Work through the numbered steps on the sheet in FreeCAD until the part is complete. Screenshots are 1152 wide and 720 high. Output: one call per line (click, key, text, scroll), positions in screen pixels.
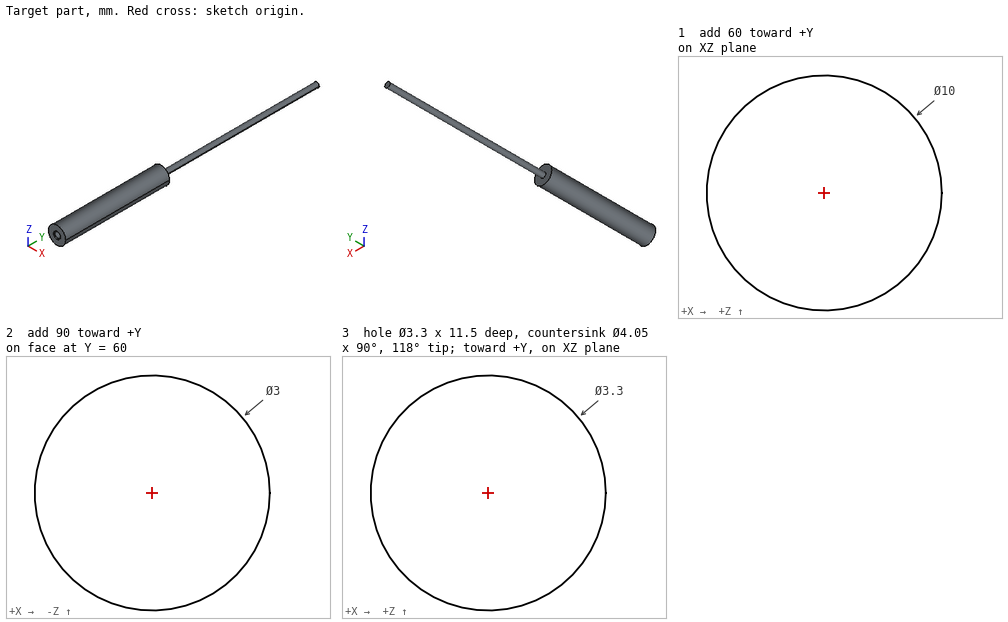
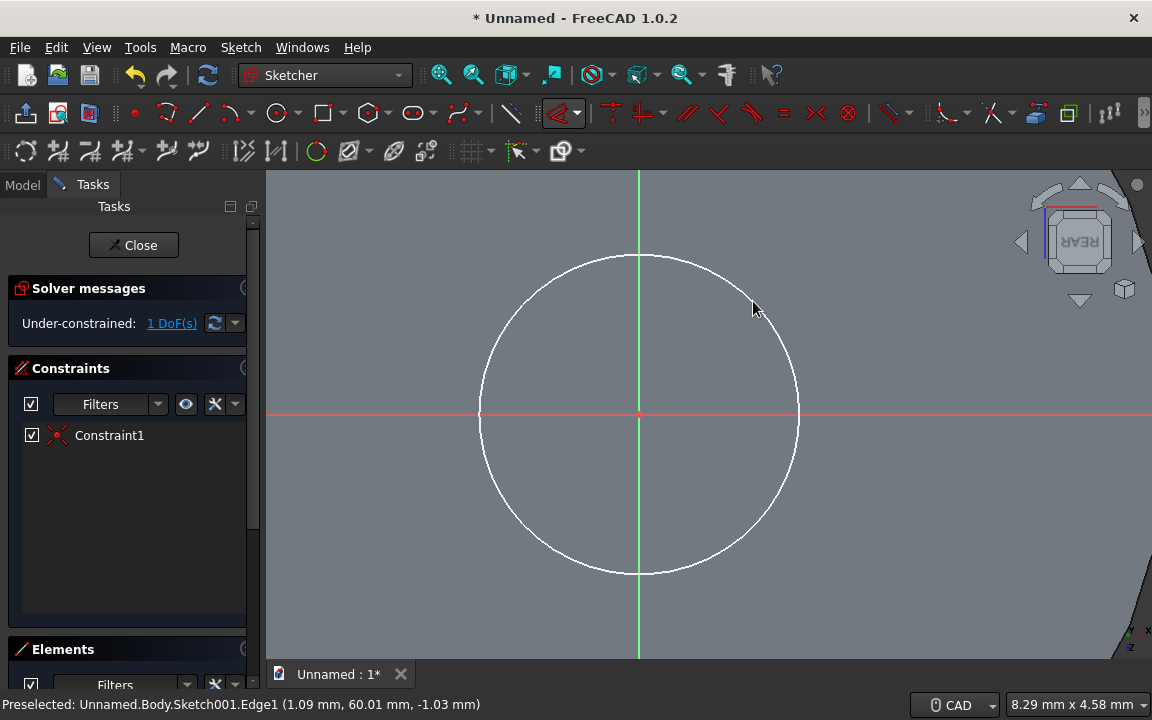
click(752, 301)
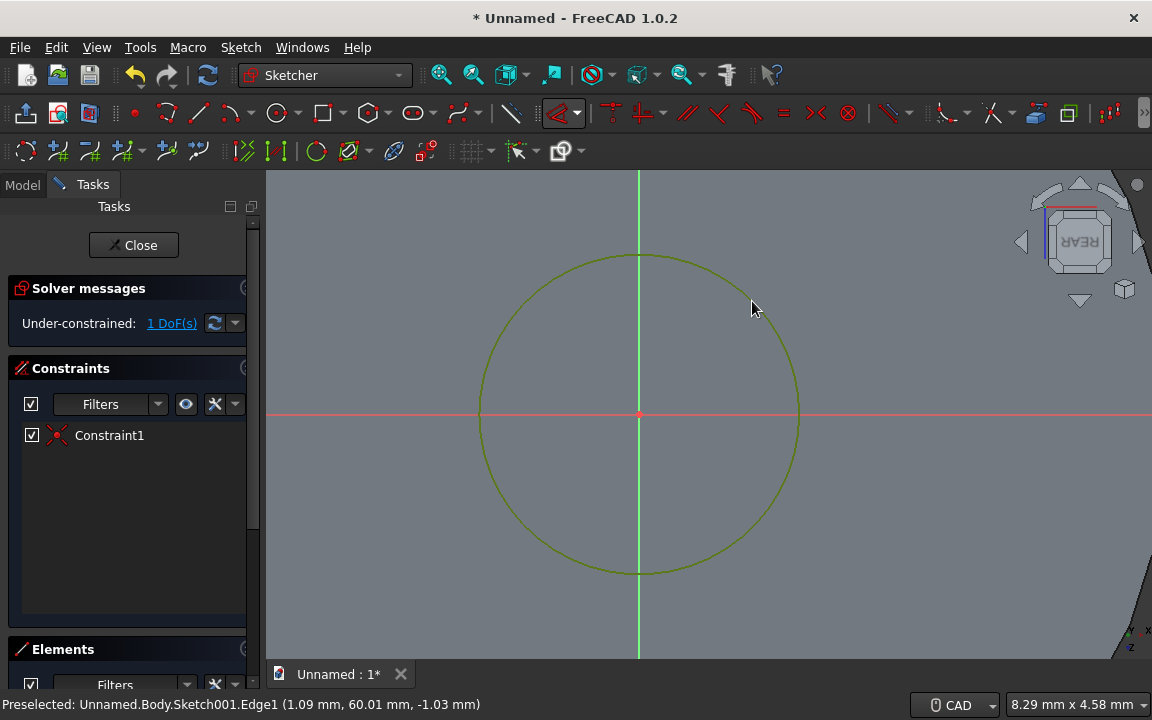
click(580, 114)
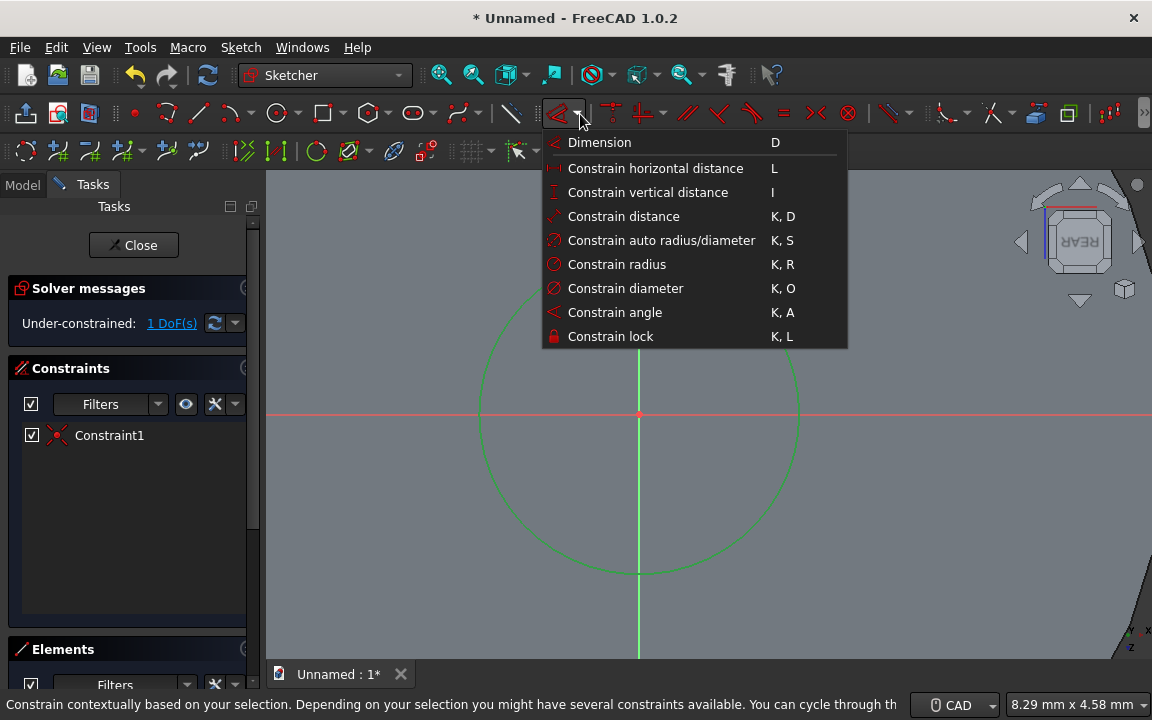
click(695, 288)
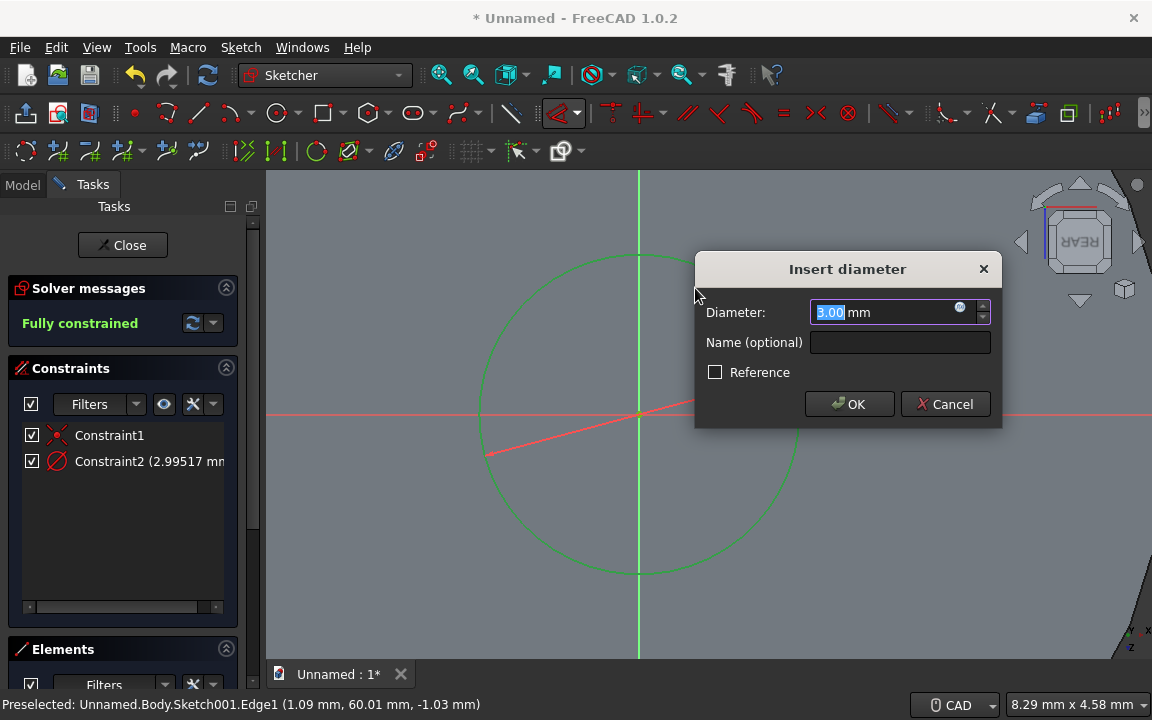
text(3)
key(Return)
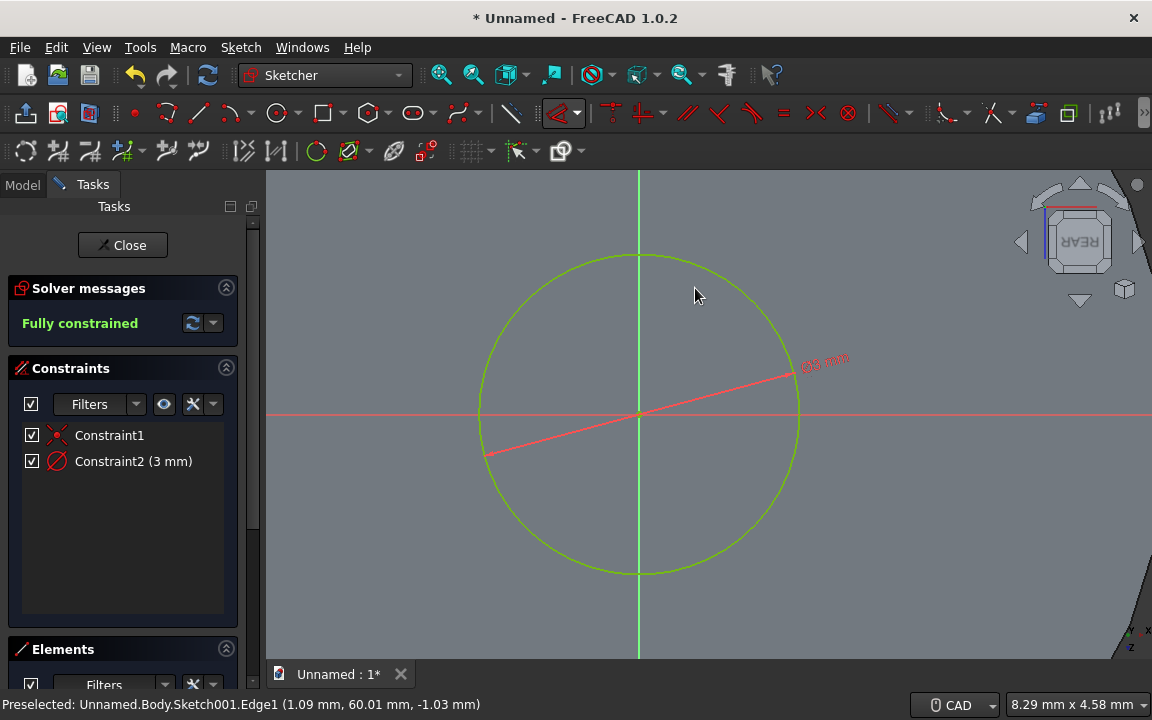
click(123, 245)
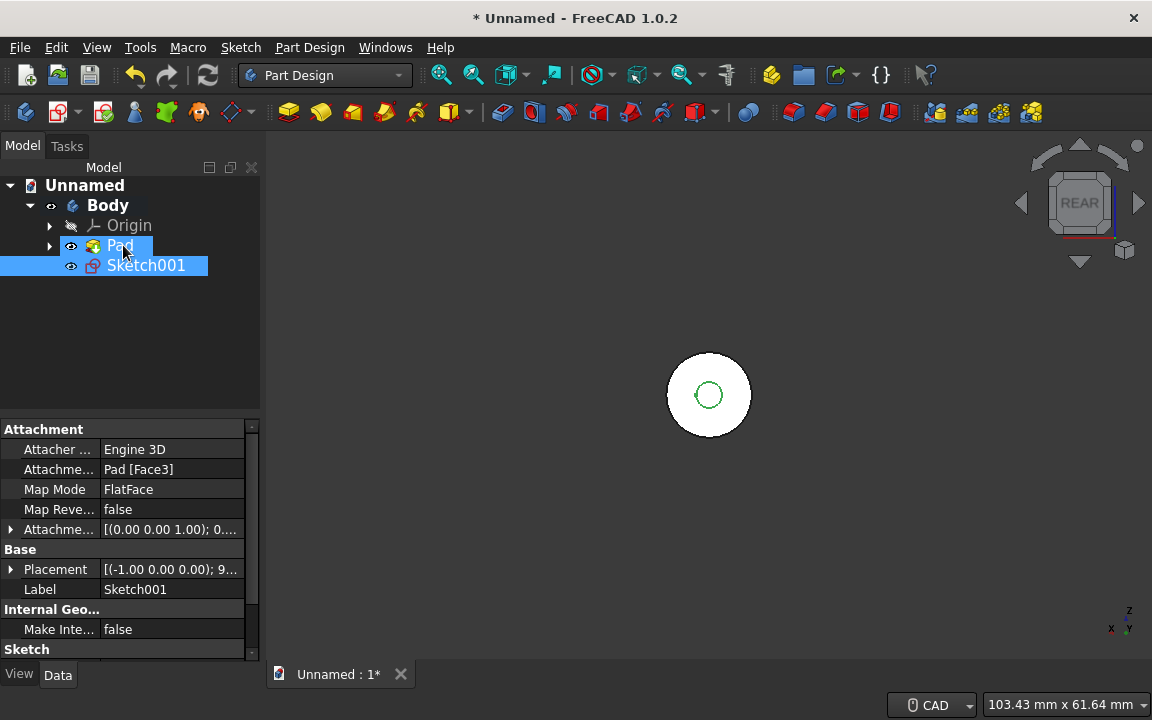
click(290, 112)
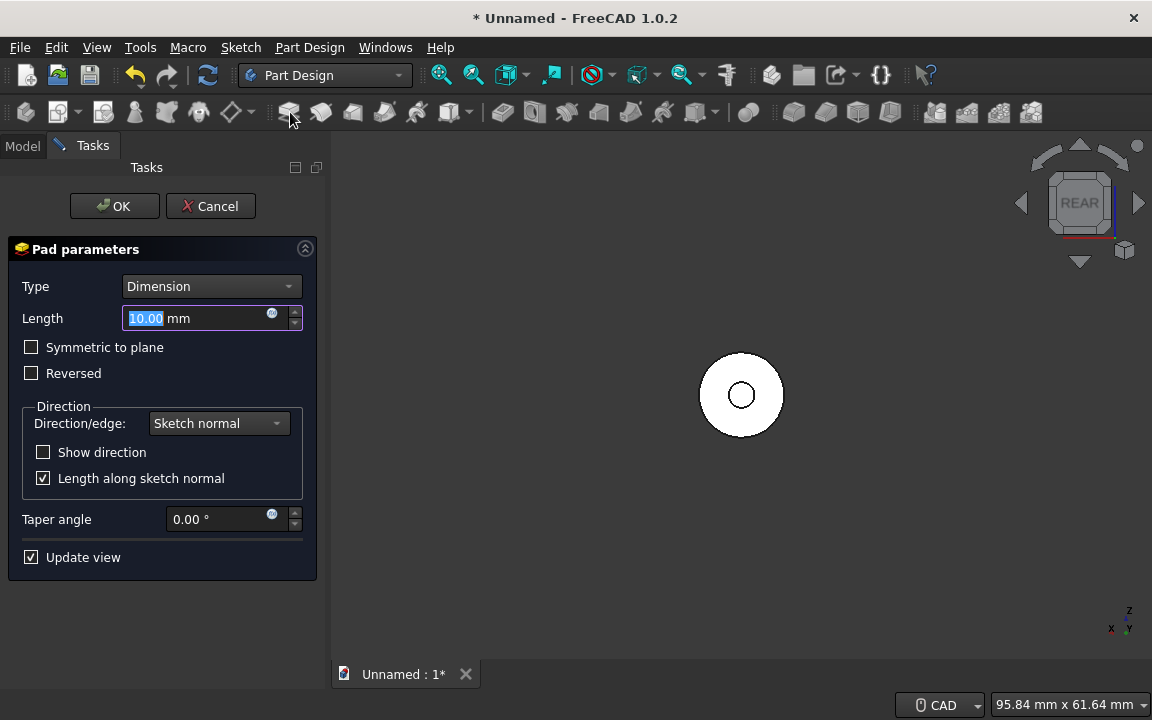
text(90)
key(Tab)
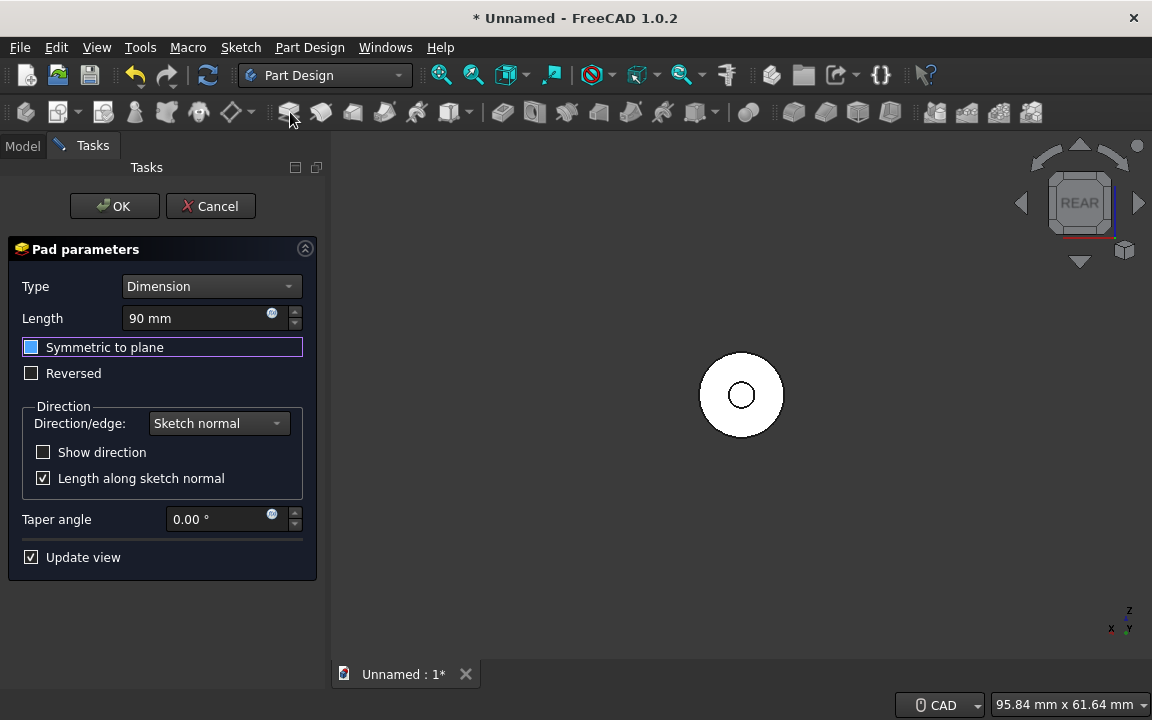
click(115, 206)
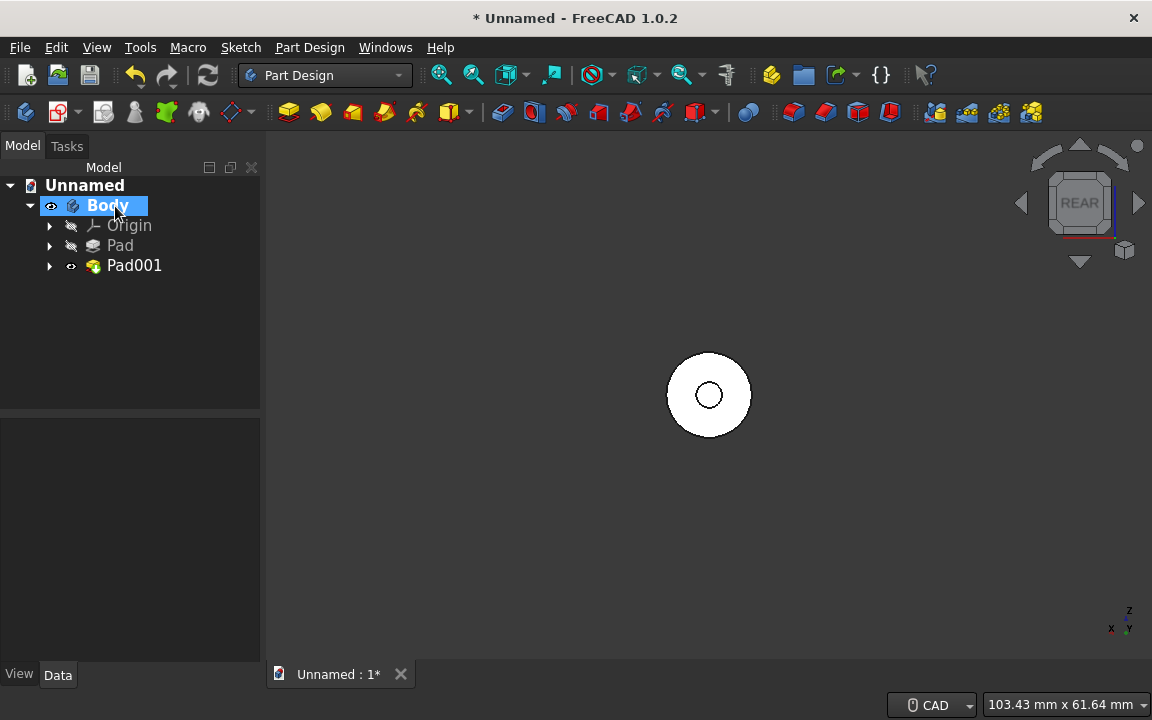
click(442, 76)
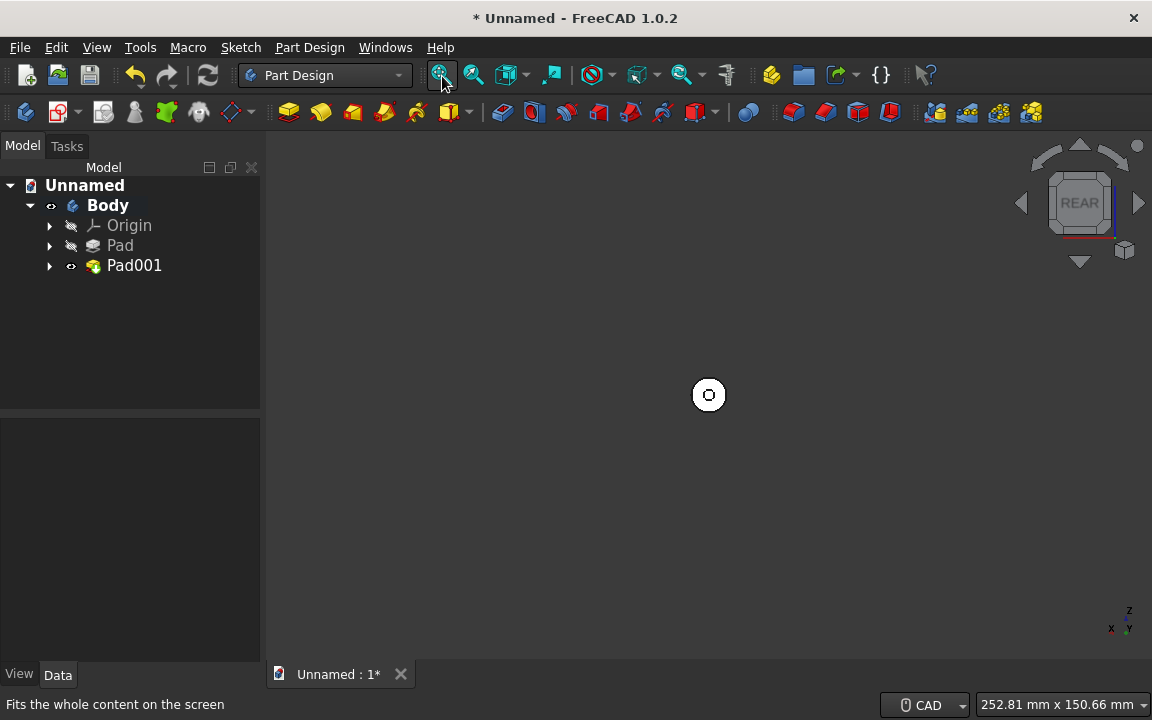
click(58, 112)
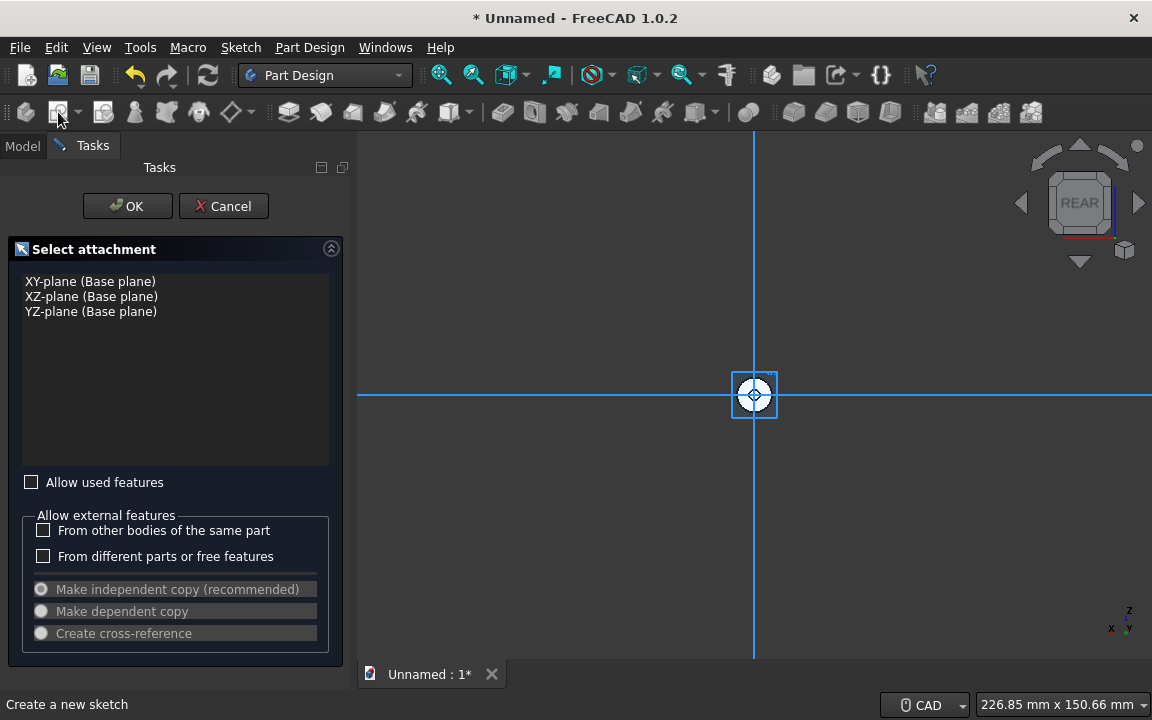
click(82, 296)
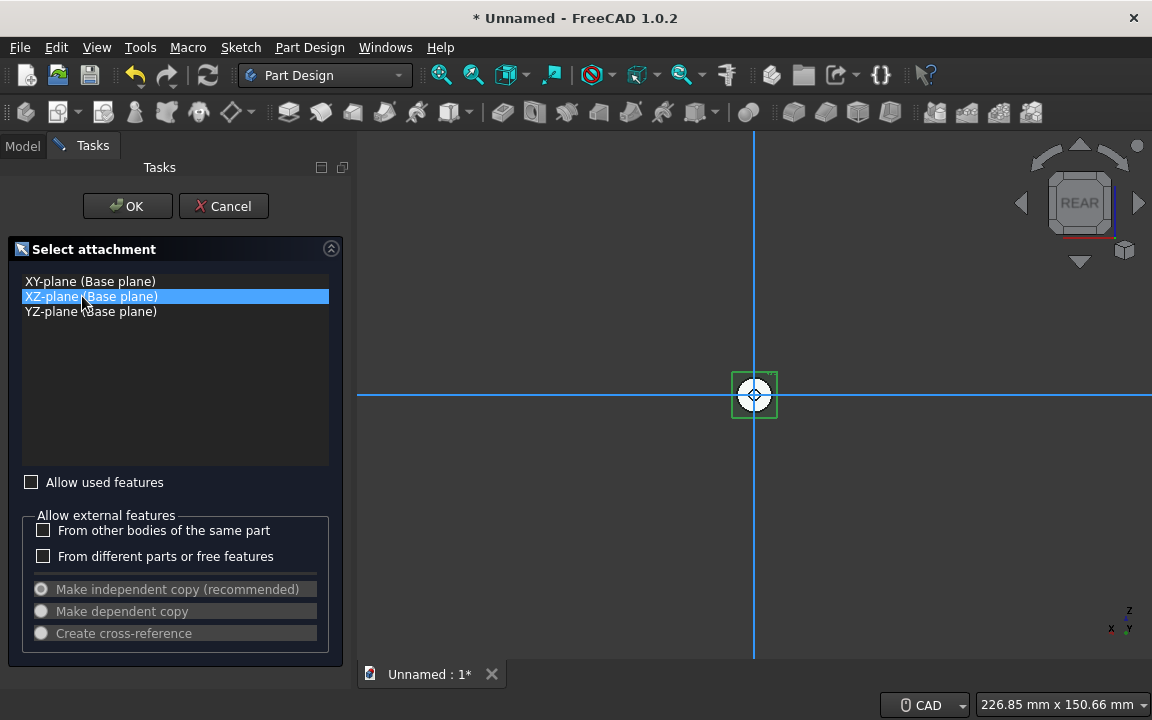
click(128, 206)